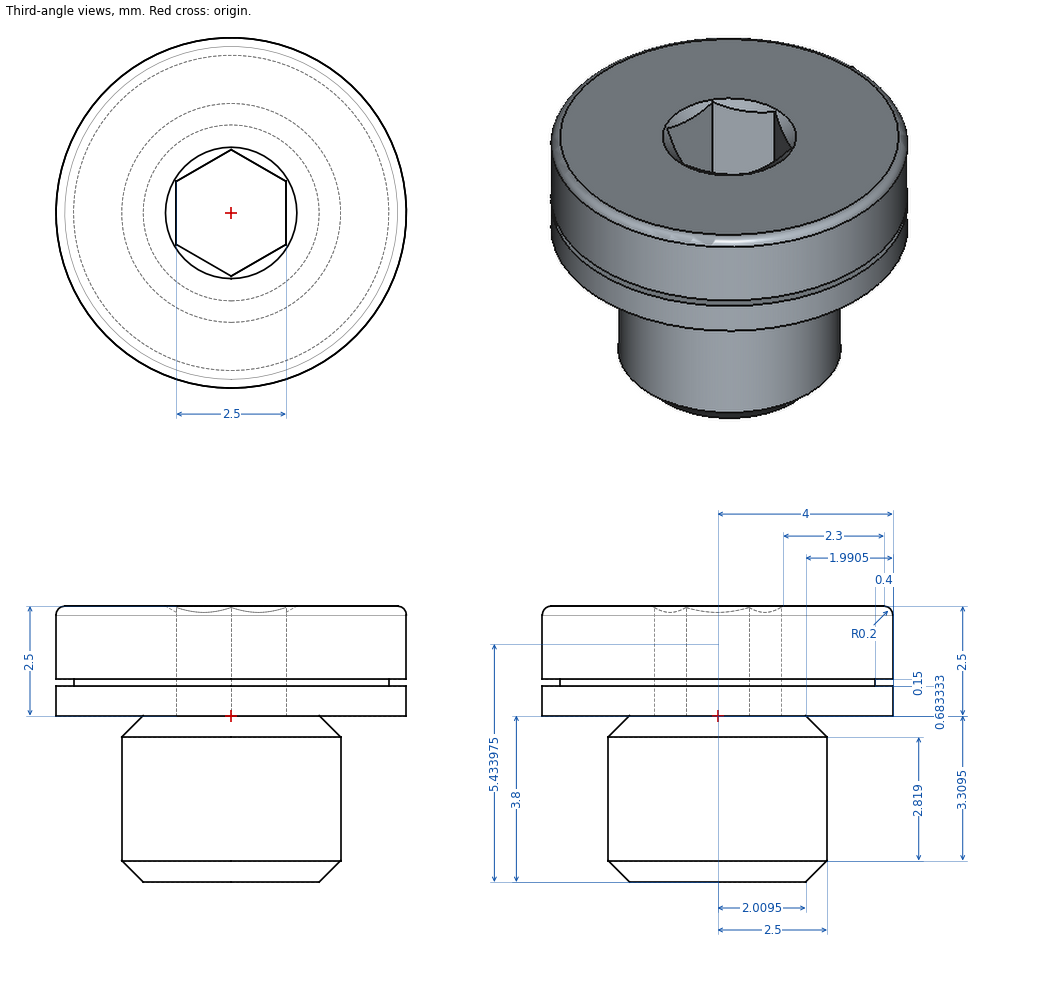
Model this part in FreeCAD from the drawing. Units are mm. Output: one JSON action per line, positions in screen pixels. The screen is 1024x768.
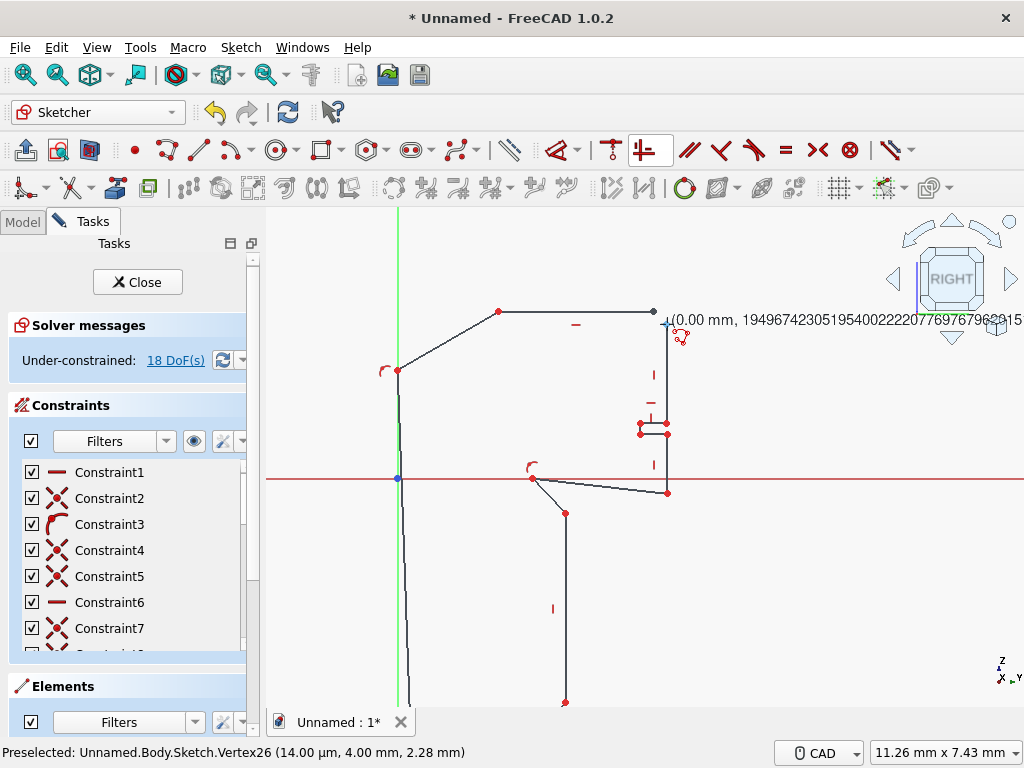
{"action": "key", "text": "g 3 a"}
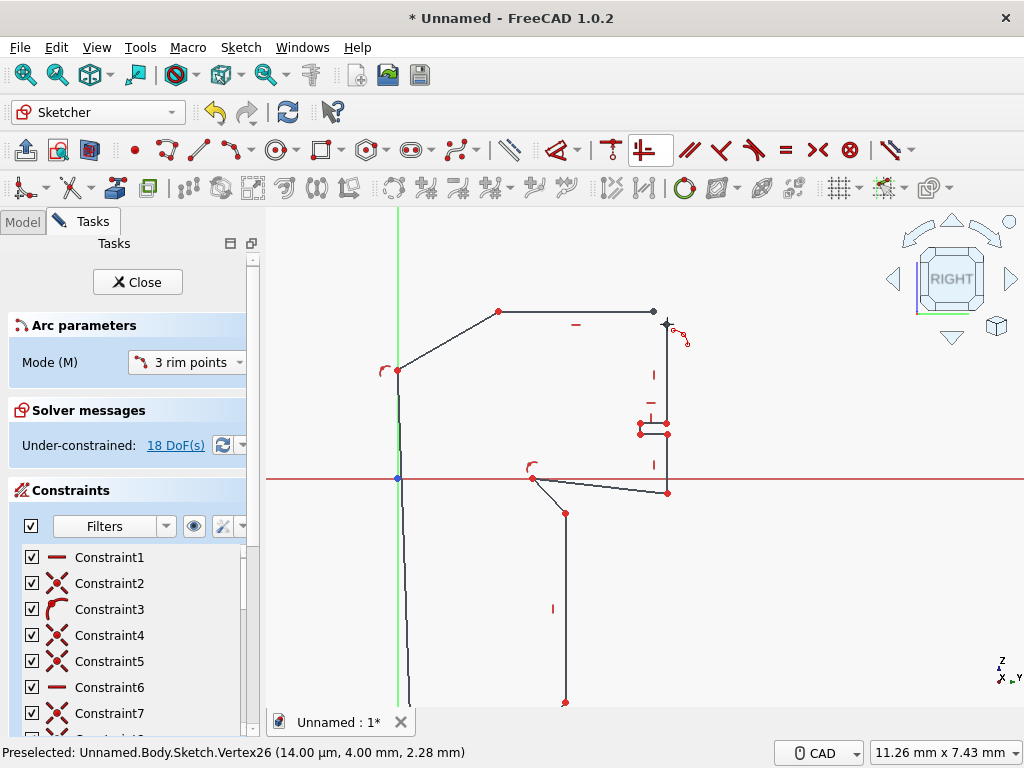
{"action": "left_click", "coordinate": [667, 325]}
{"action": "left_click", "coordinate": [654, 312]}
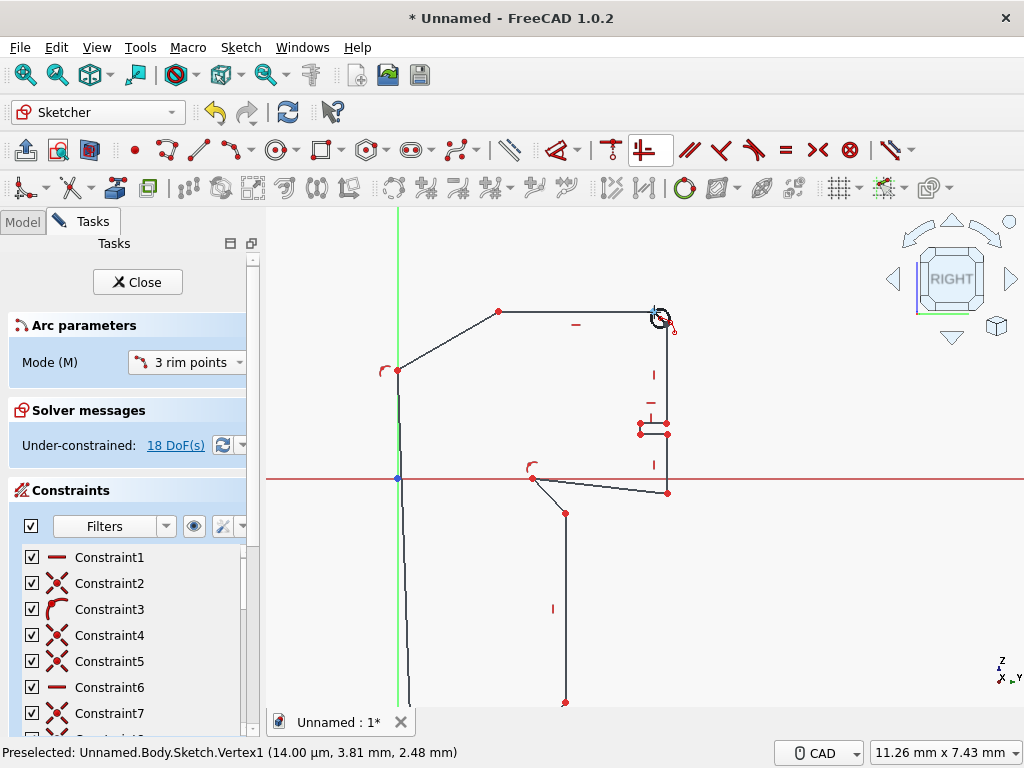
{"action": "scroll", "coordinate": [663, 314], "scroll_direction": "up", "scroll_amount": 7}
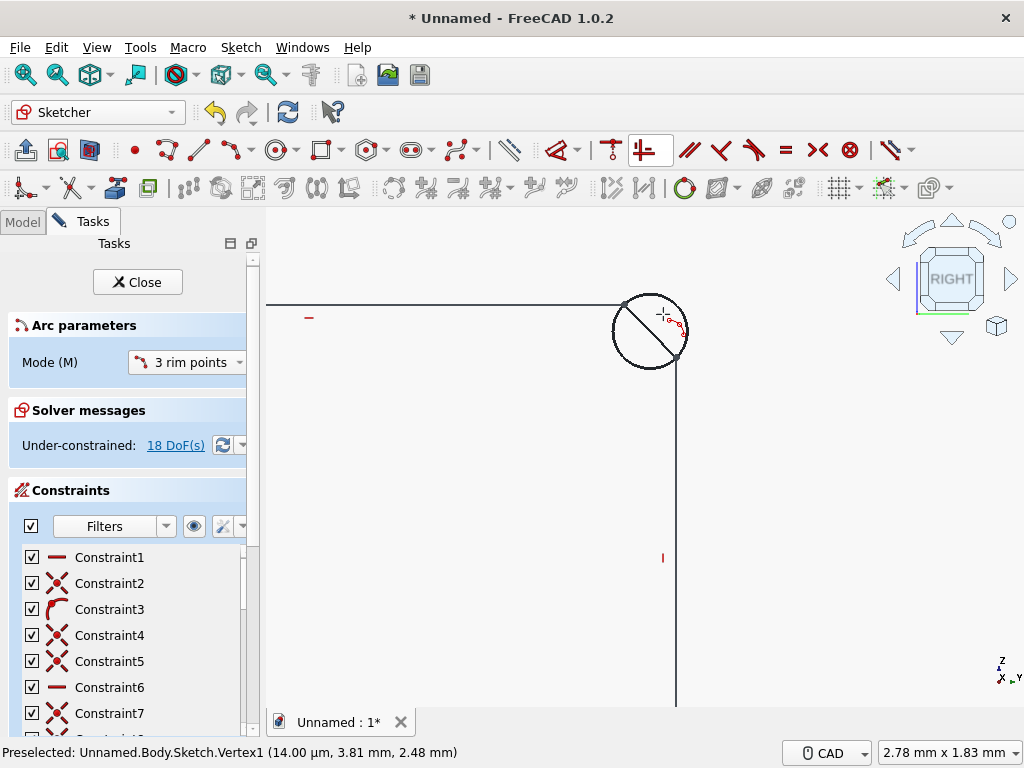
{"action": "left_click", "coordinate": [661, 315]}
{"action": "key", "text": "Escape"}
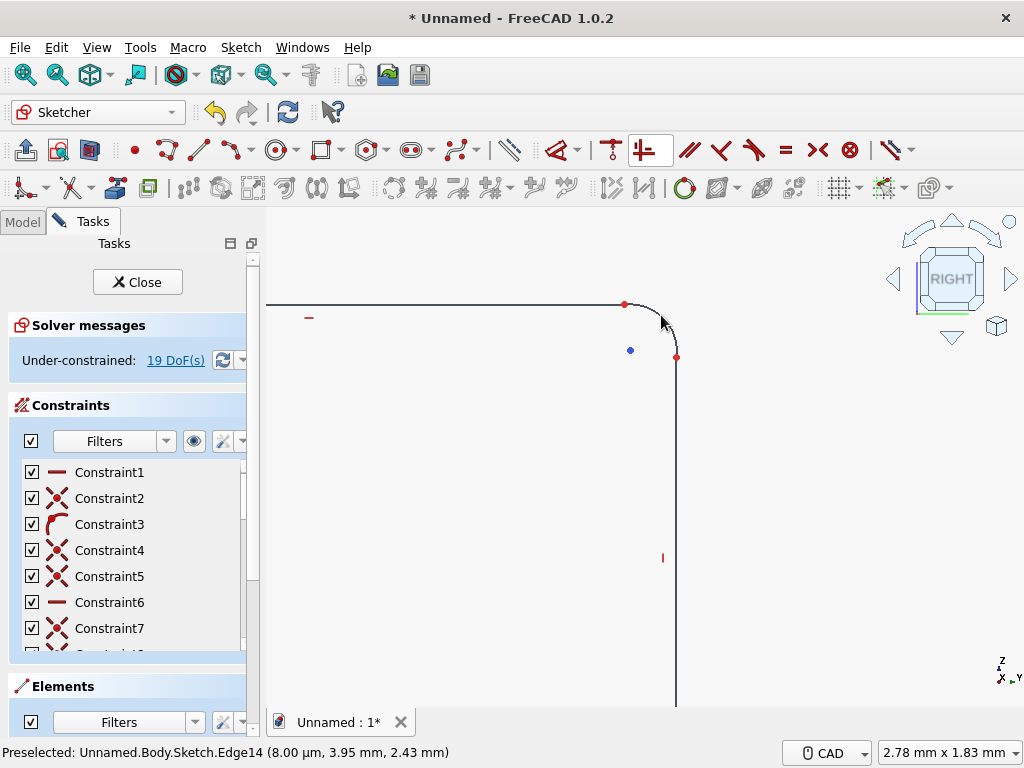
{"action": "scroll", "coordinate": [665, 318], "scroll_direction": "down", "scroll_amount": 9}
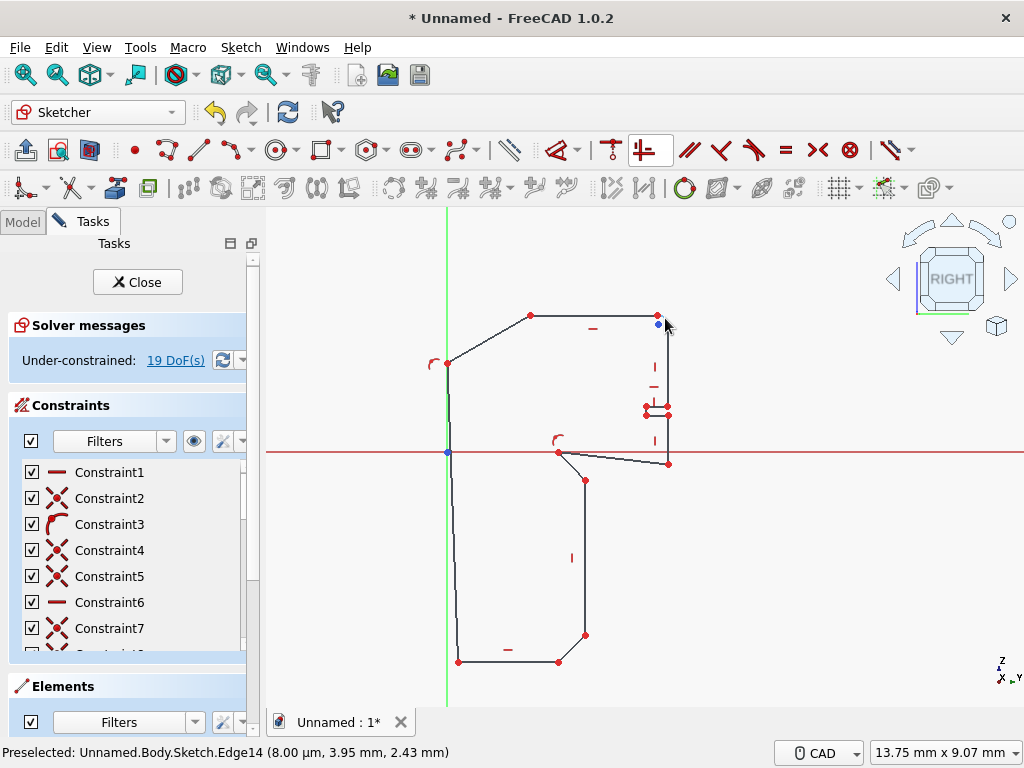
{"action": "left_click", "coordinate": [627, 316]}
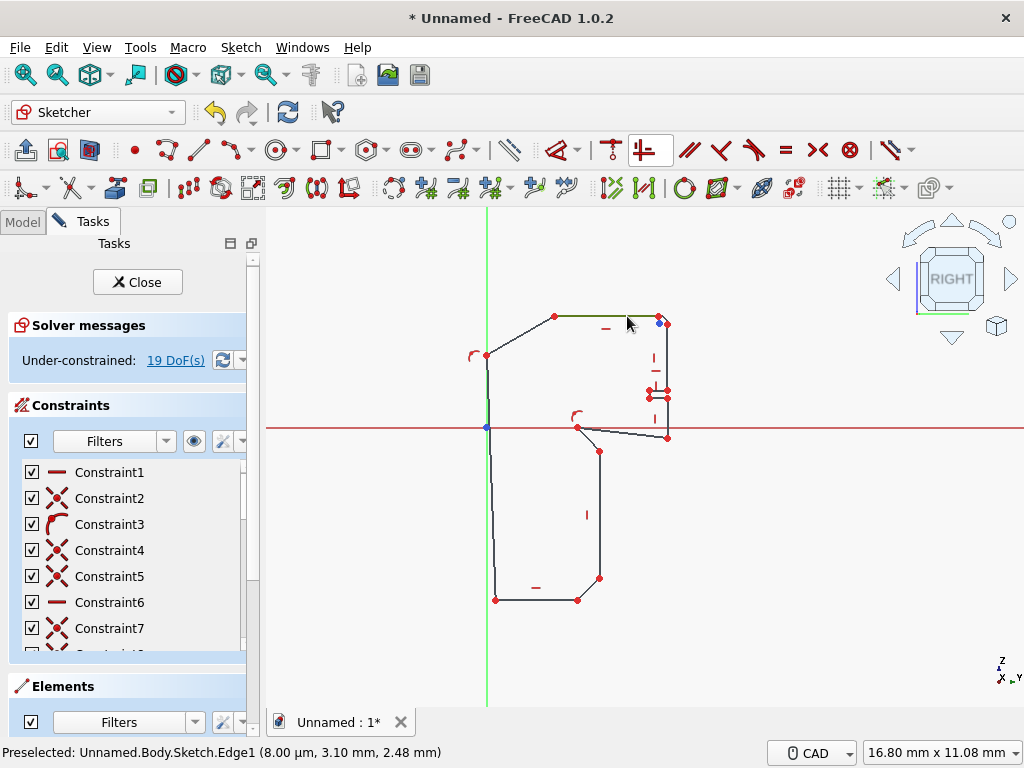
{"action": "scroll", "coordinate": [665, 318], "scroll_direction": "up", "scroll_amount": 4}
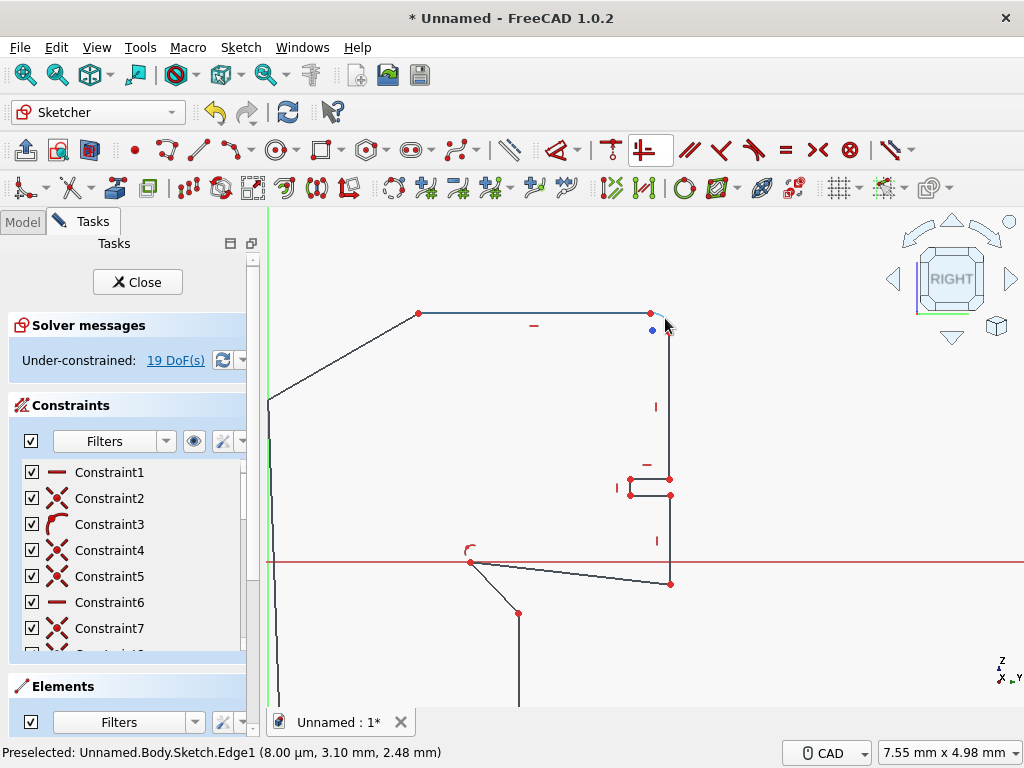
{"action": "left_click", "coordinate": [665, 318]}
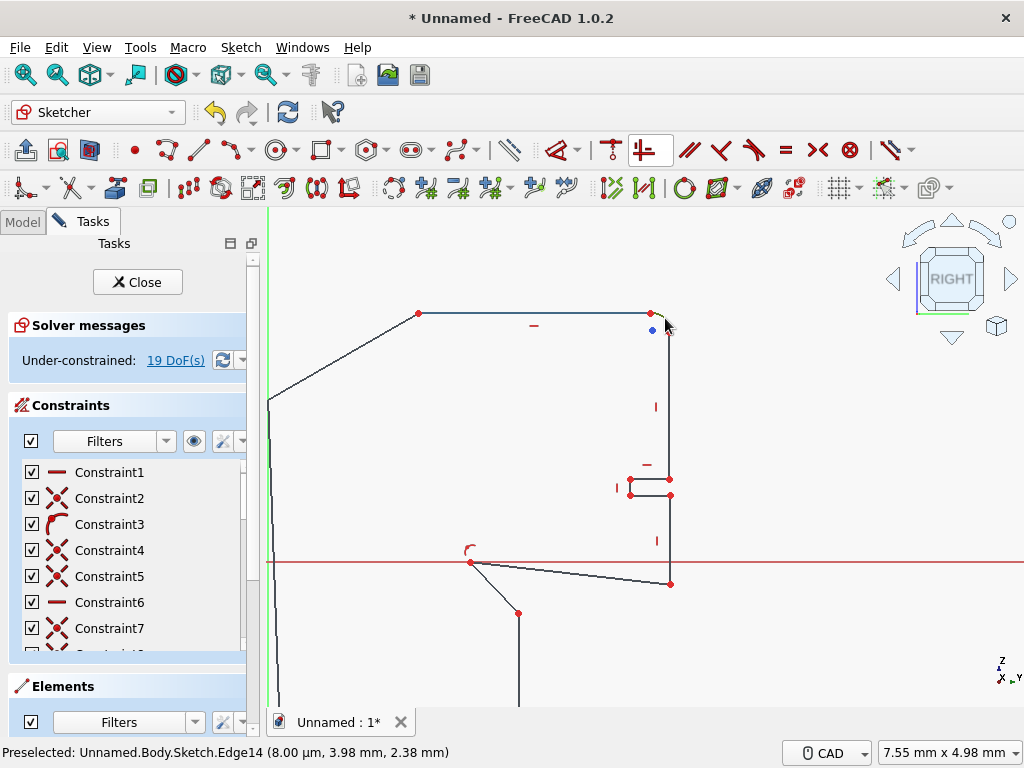
{"action": "left_click", "coordinate": [754, 150]}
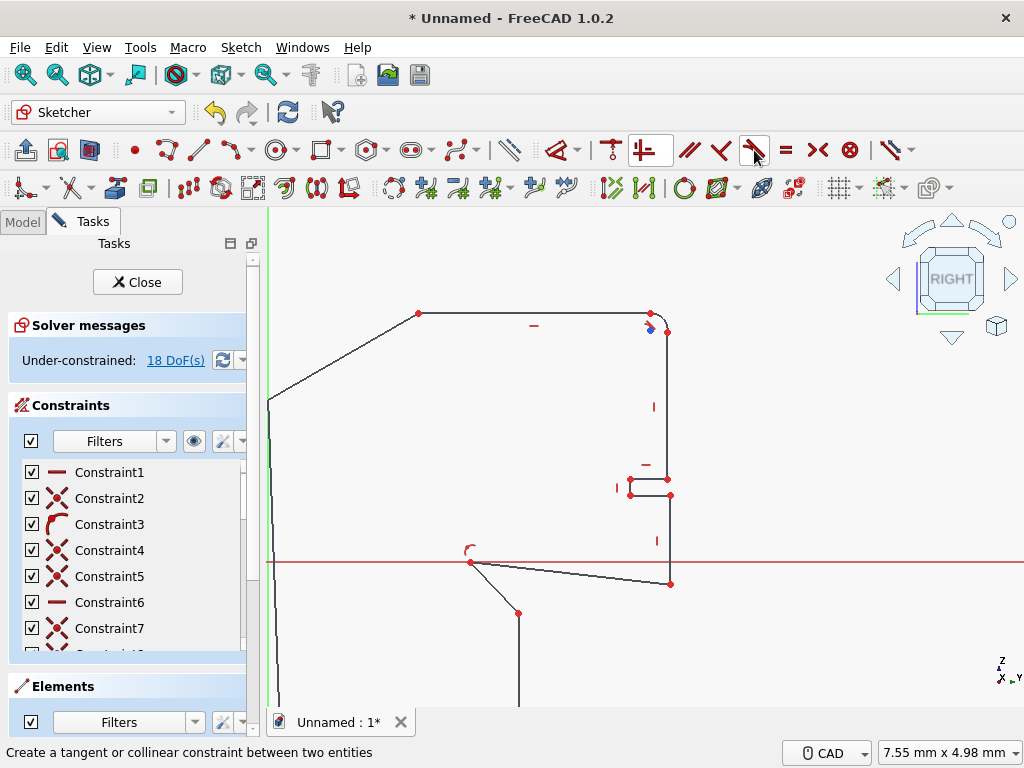
{"action": "left_click", "coordinate": [667, 435]}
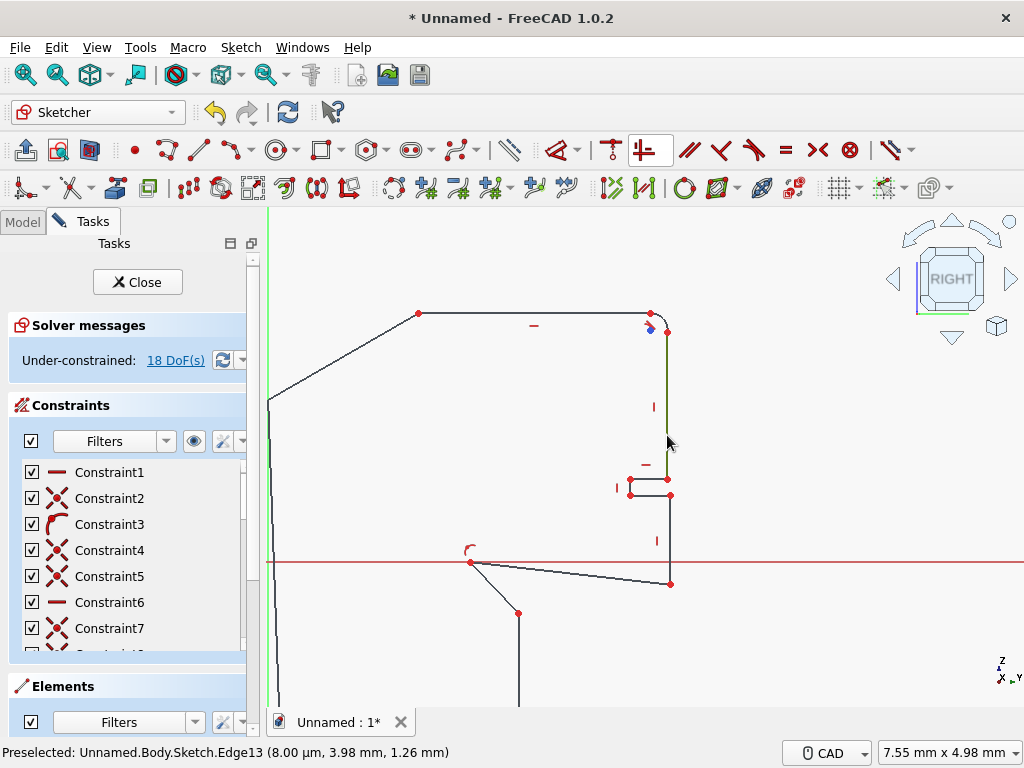
{"action": "left_click", "coordinate": [664, 319]}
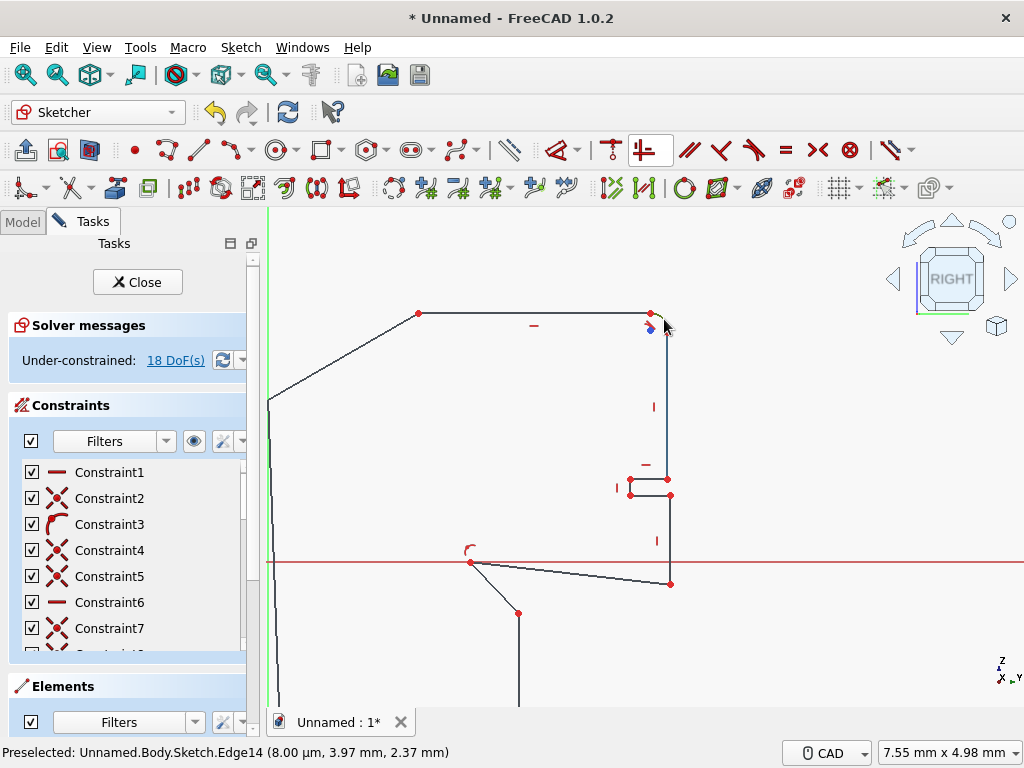
{"action": "key", "text": "t"}